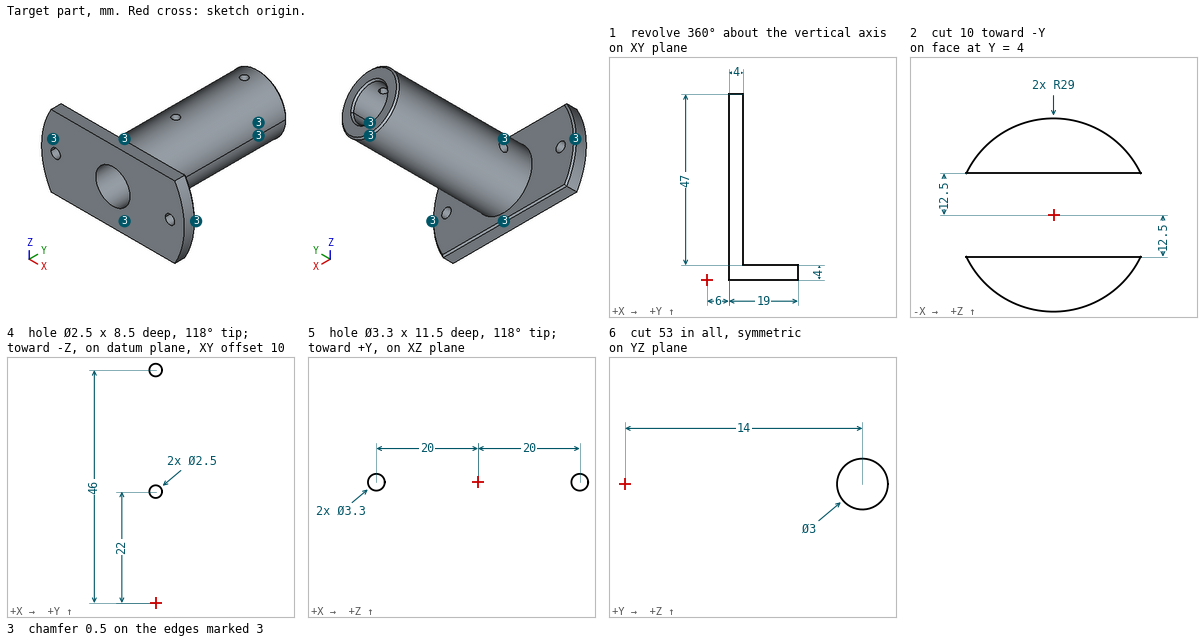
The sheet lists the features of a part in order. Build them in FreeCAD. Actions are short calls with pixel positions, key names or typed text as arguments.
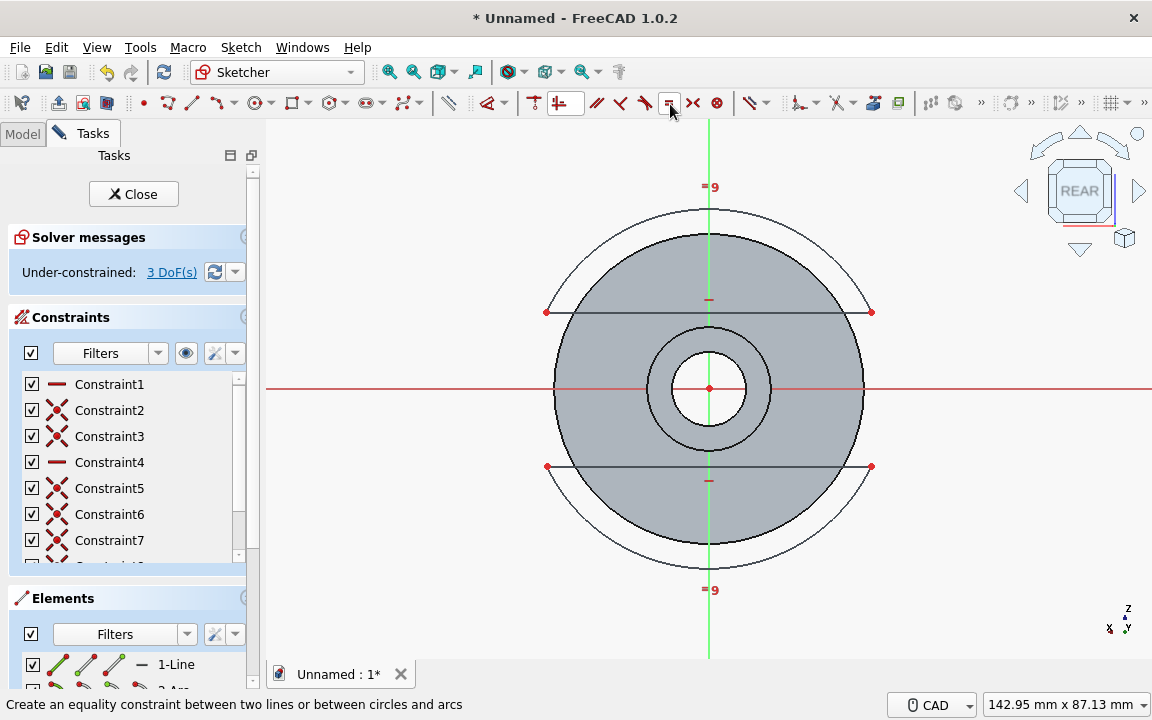
click(488, 104)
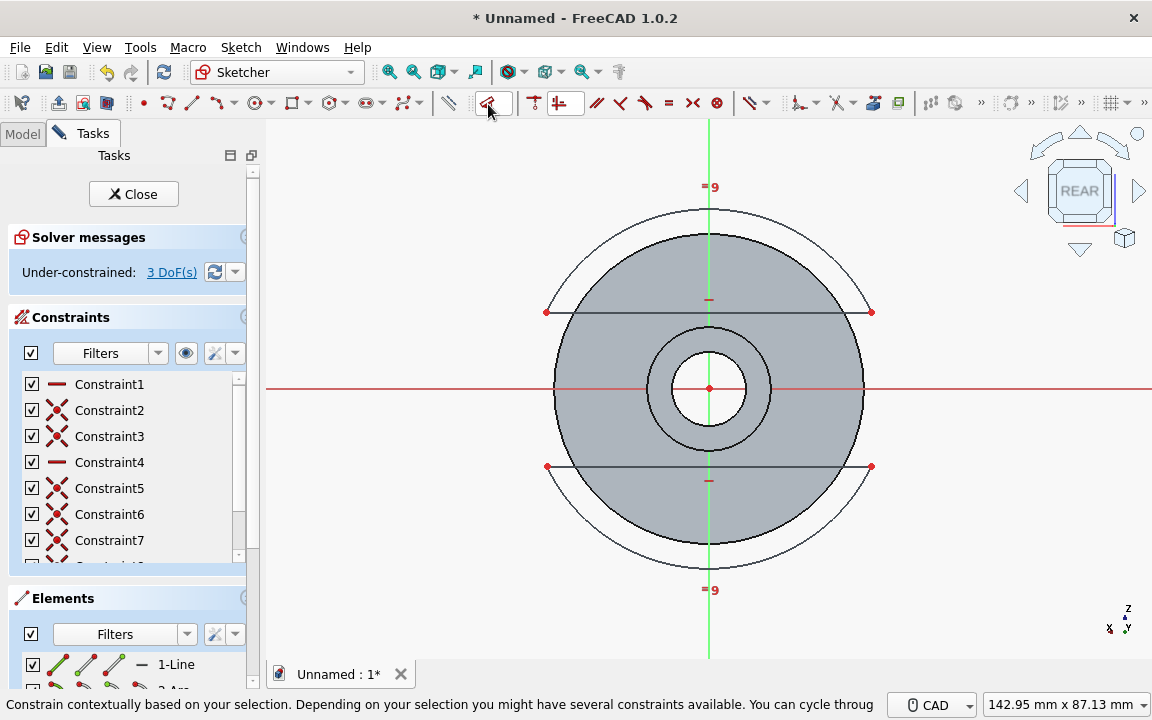
click(788, 227)
click(802, 198)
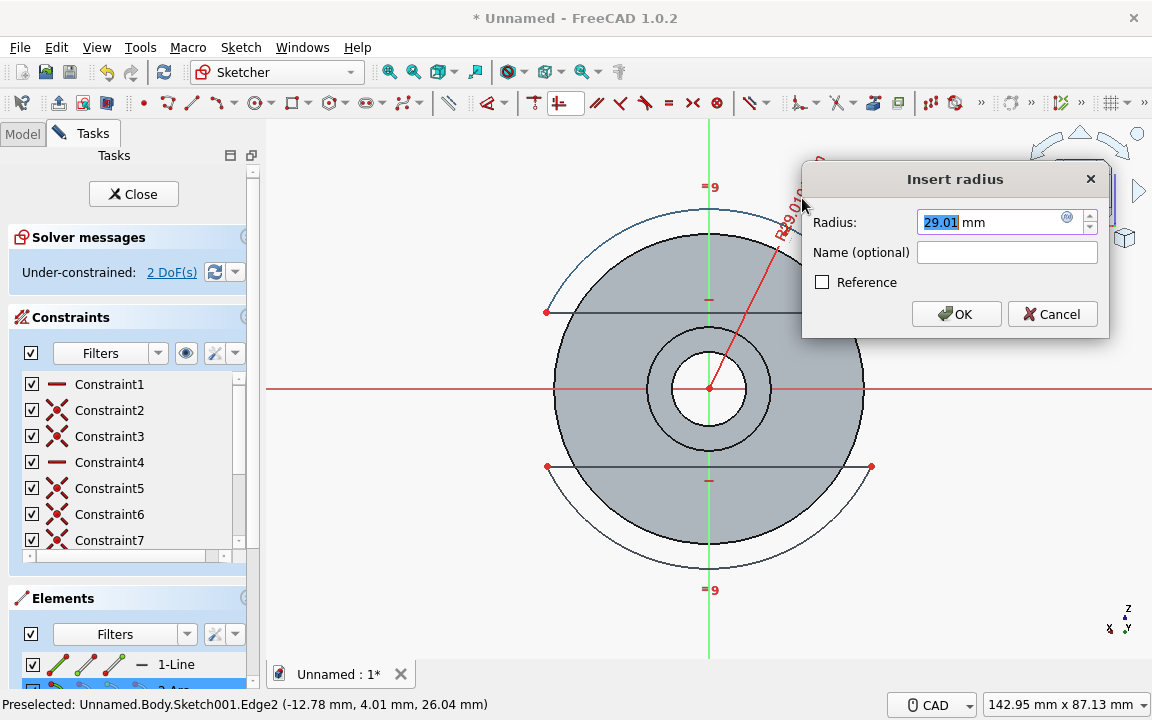
text(29)
key(Return)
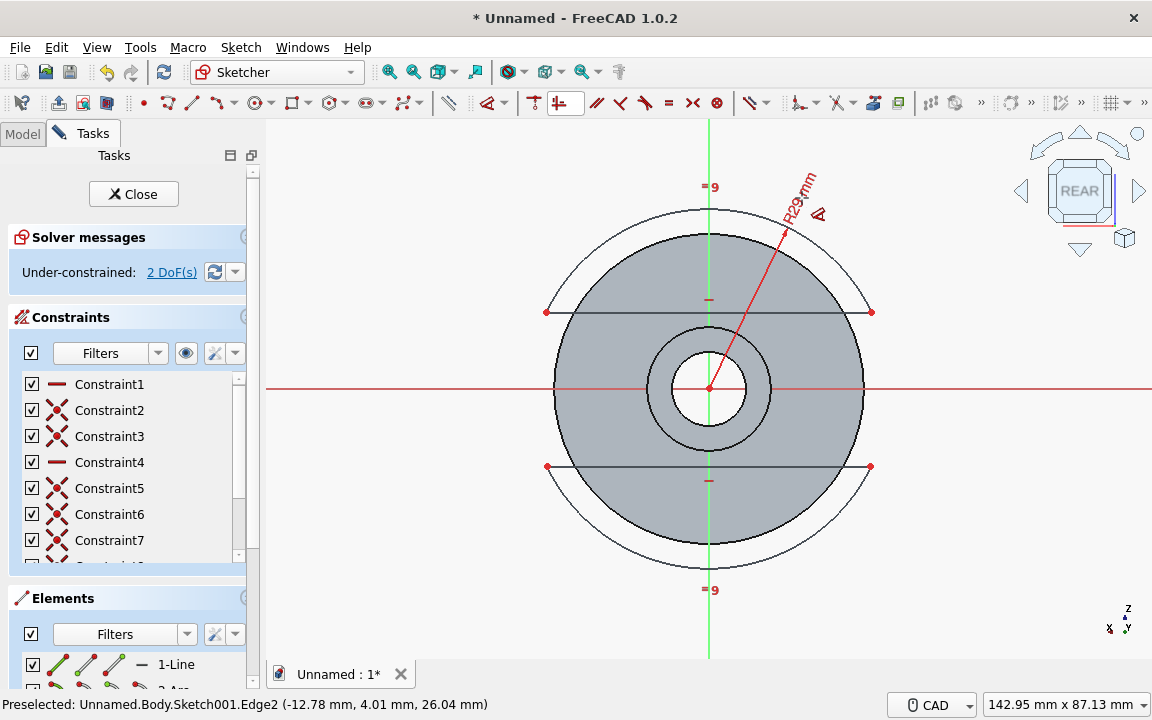
click(546, 313)
click(512, 351)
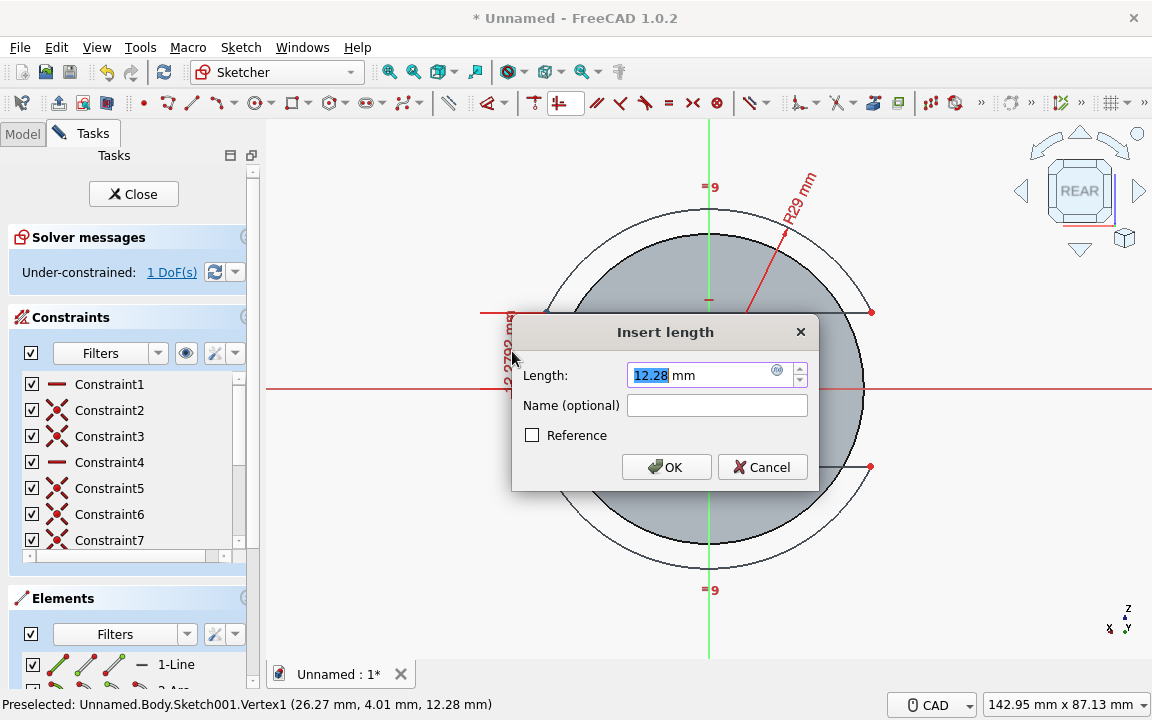
text(12.5)
key(Return)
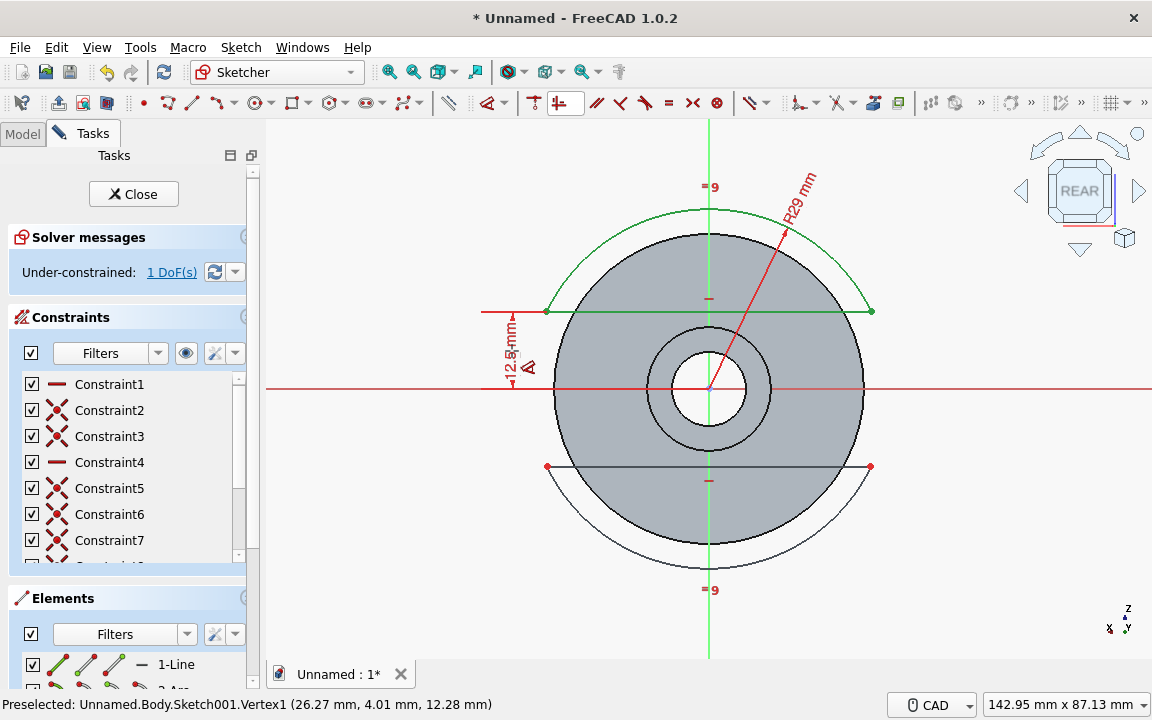
click(871, 467)
click(905, 428)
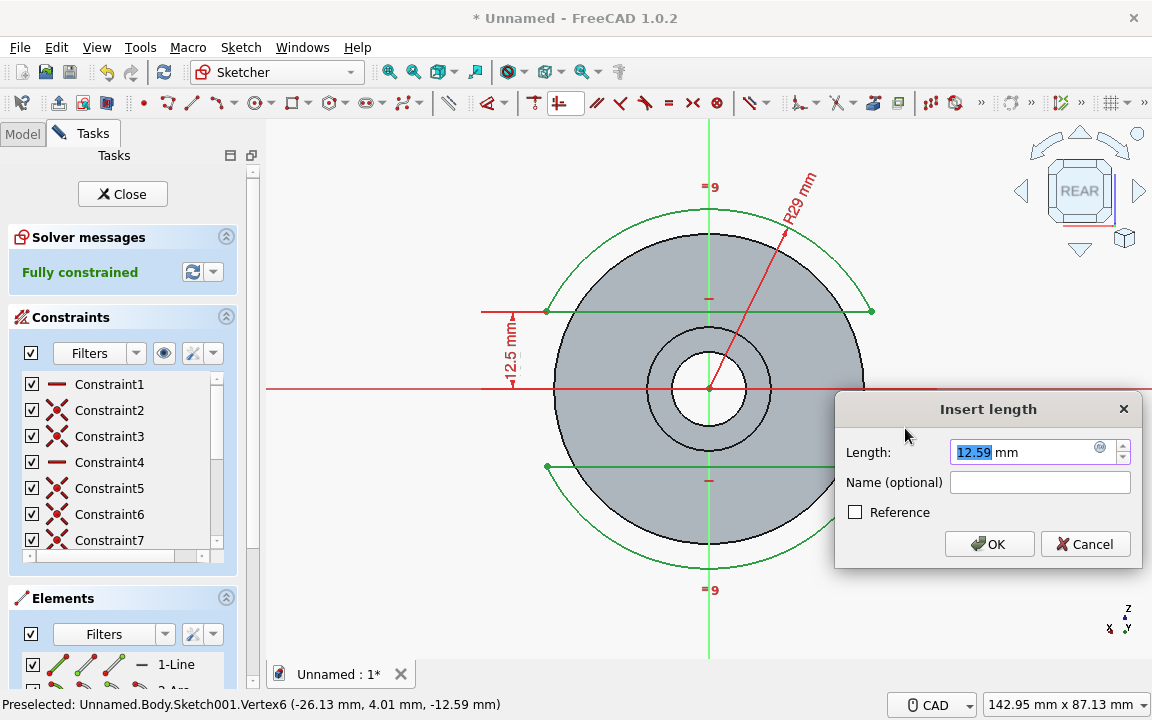
text(12.5)
key(Return)
key(Escape)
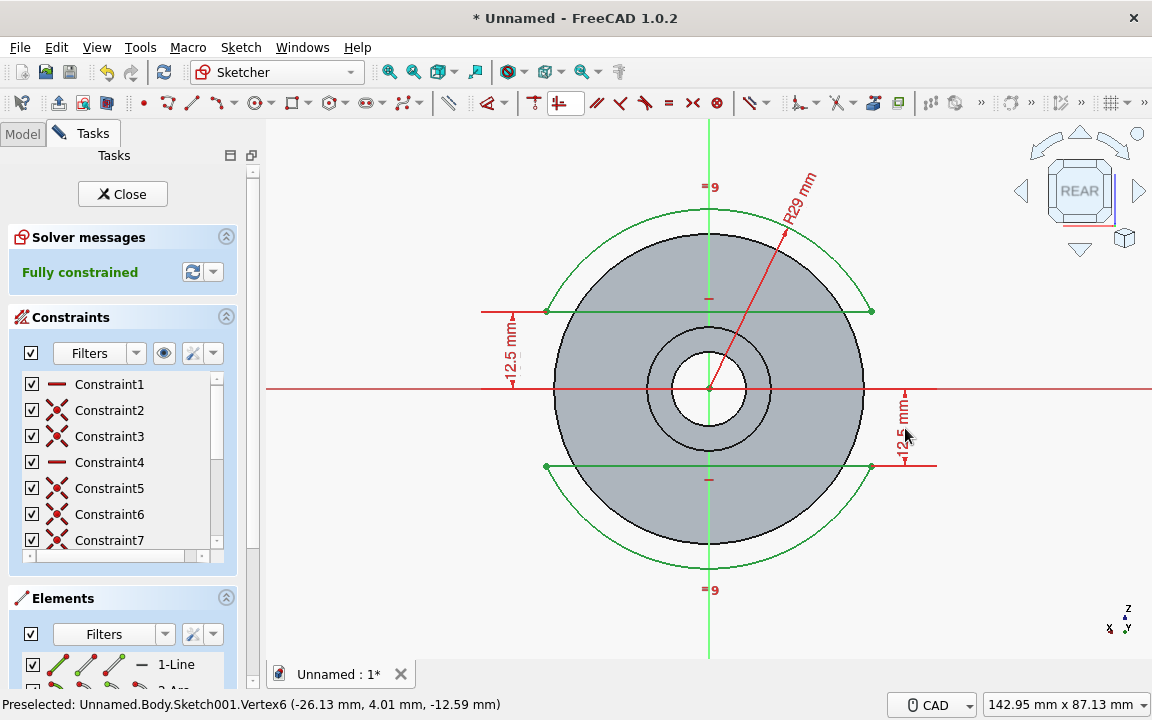
click(123, 194)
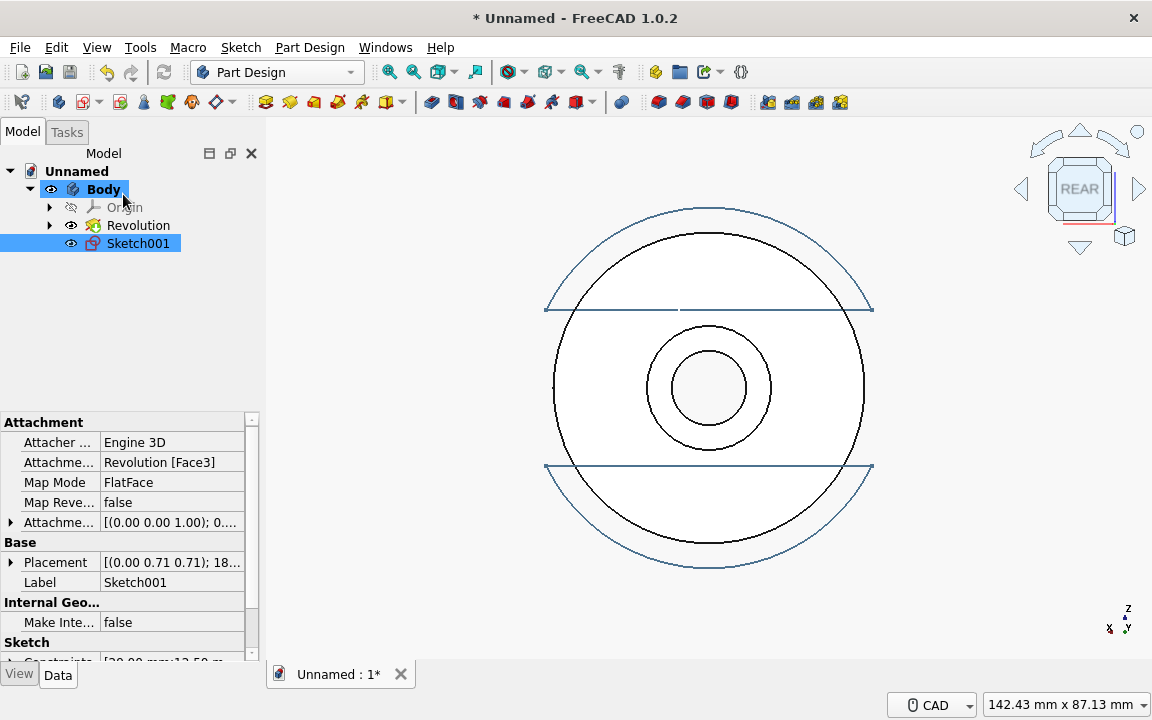
click(432, 102)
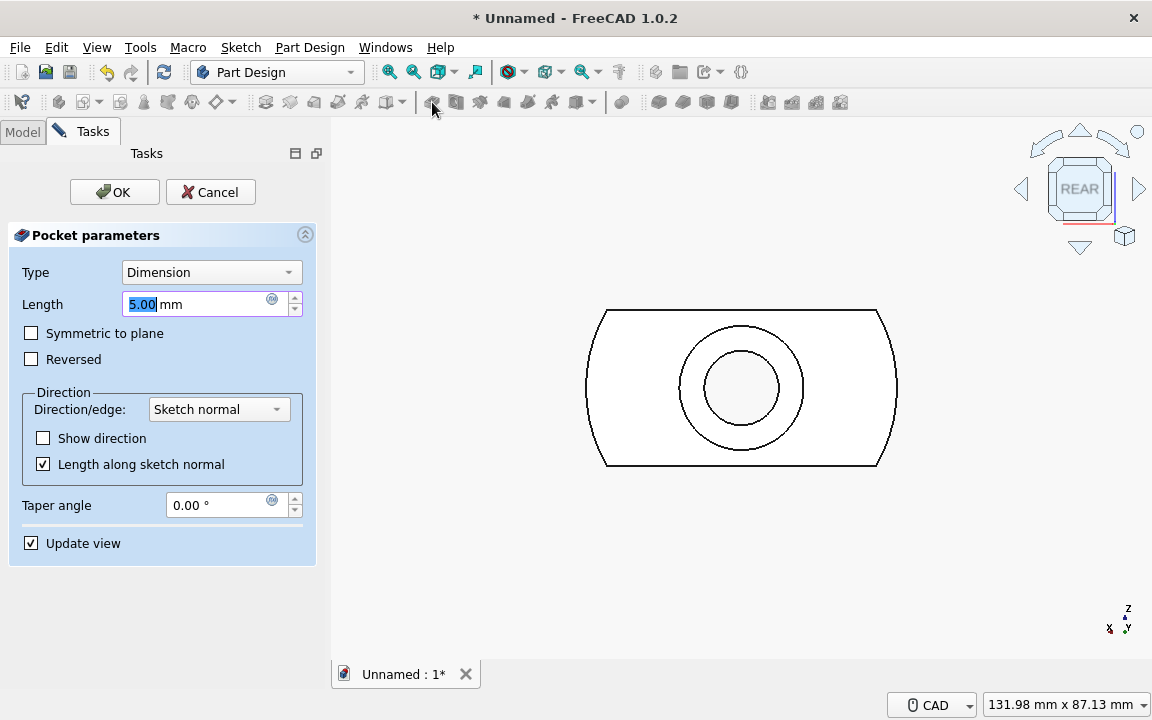
text(10)
key(Tab)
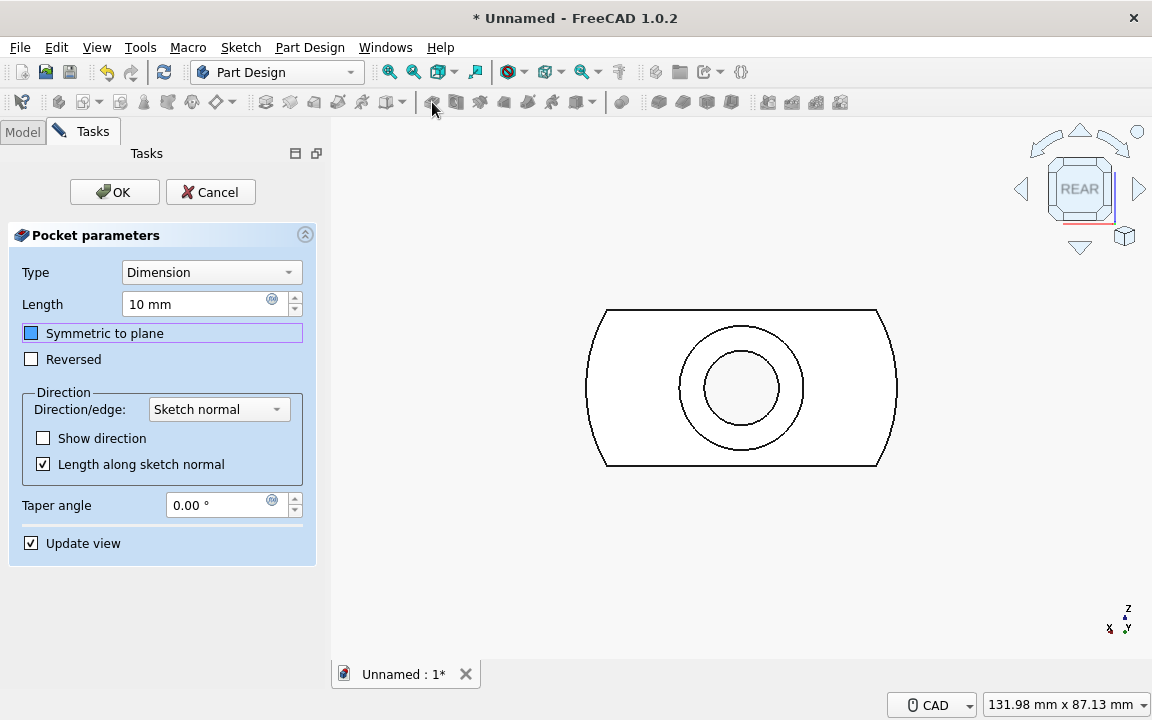
click(115, 192)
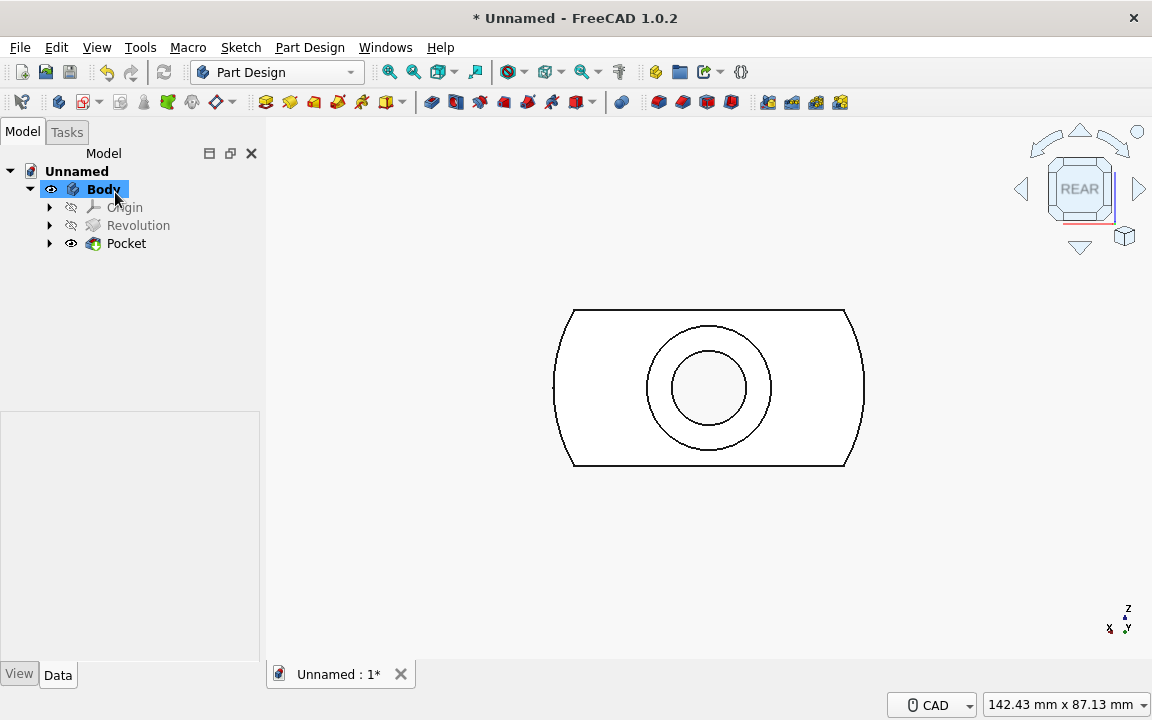
click(390, 72)